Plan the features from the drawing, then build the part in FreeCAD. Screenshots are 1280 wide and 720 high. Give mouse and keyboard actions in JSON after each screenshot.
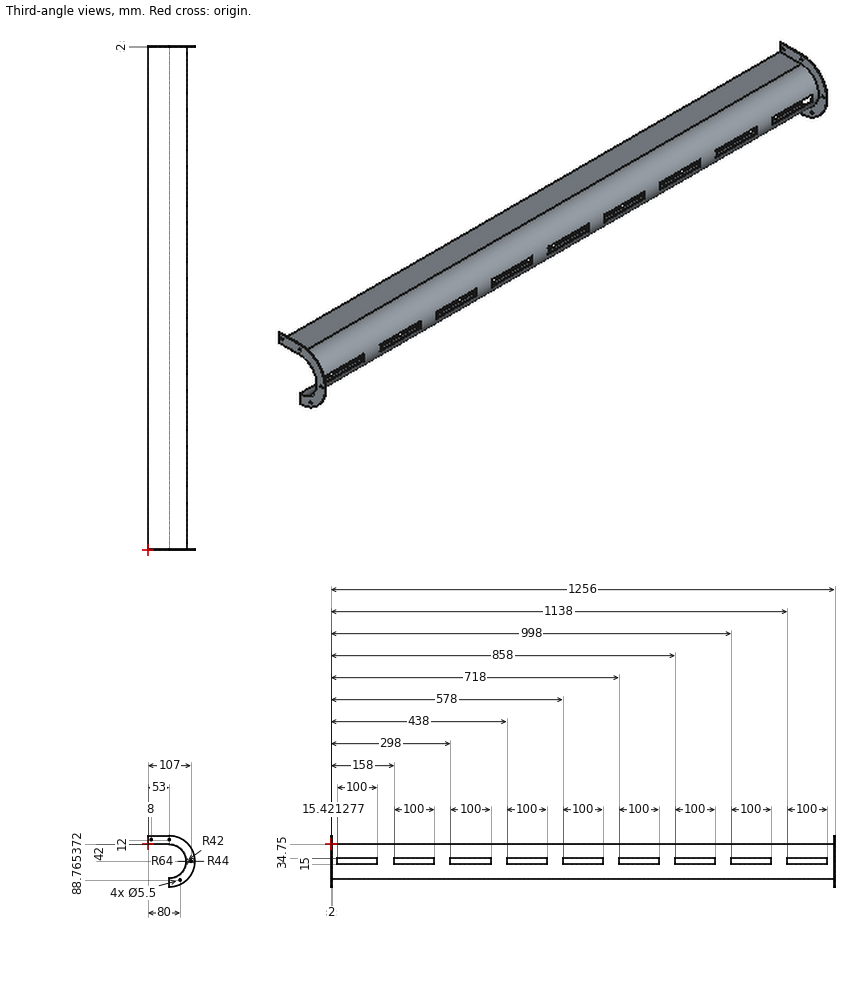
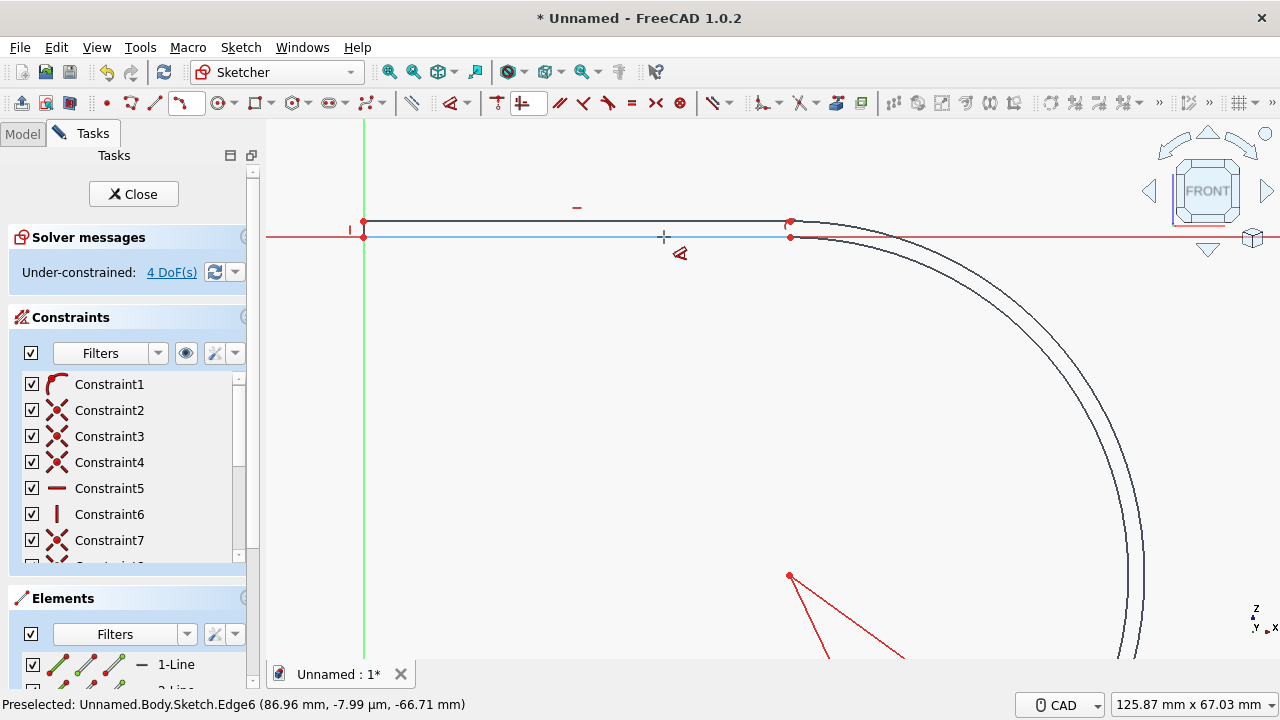
{"action": "left_click", "coordinate": [663, 237]}
{"action": "left_click", "coordinate": [577, 203]}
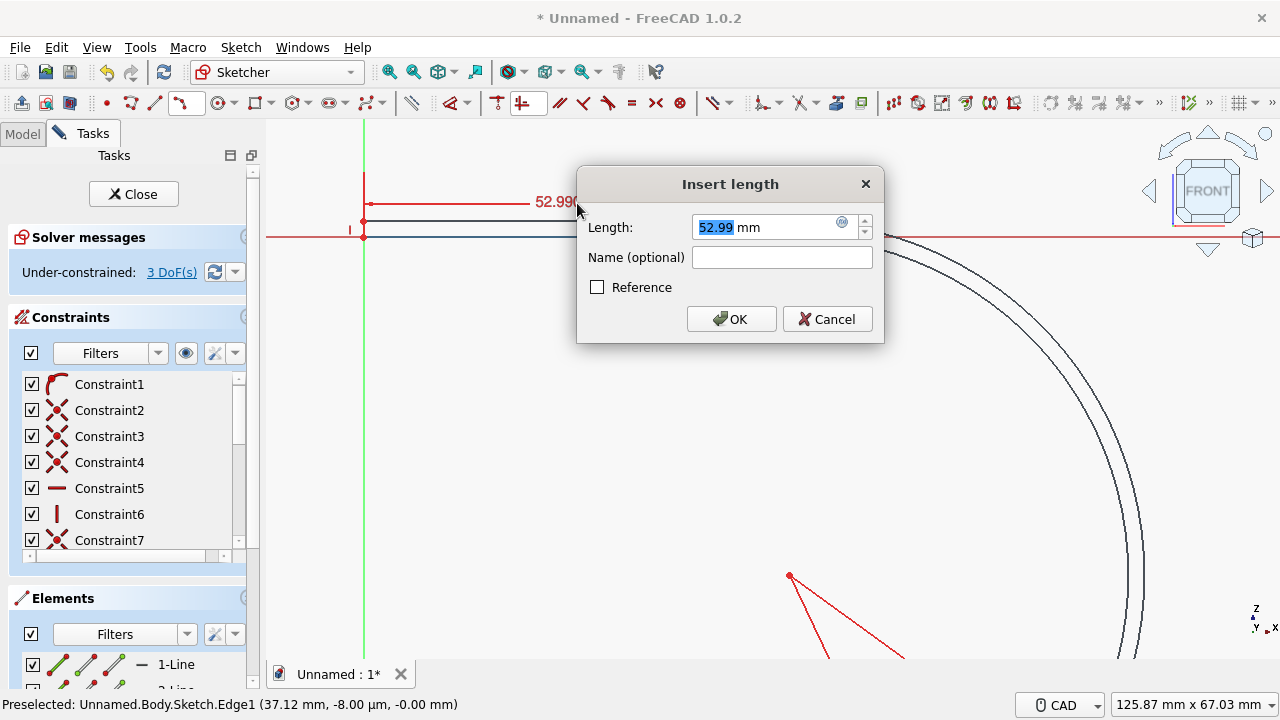
{"action": "type", "text": "53"}
{"action": "key", "text": "Return"}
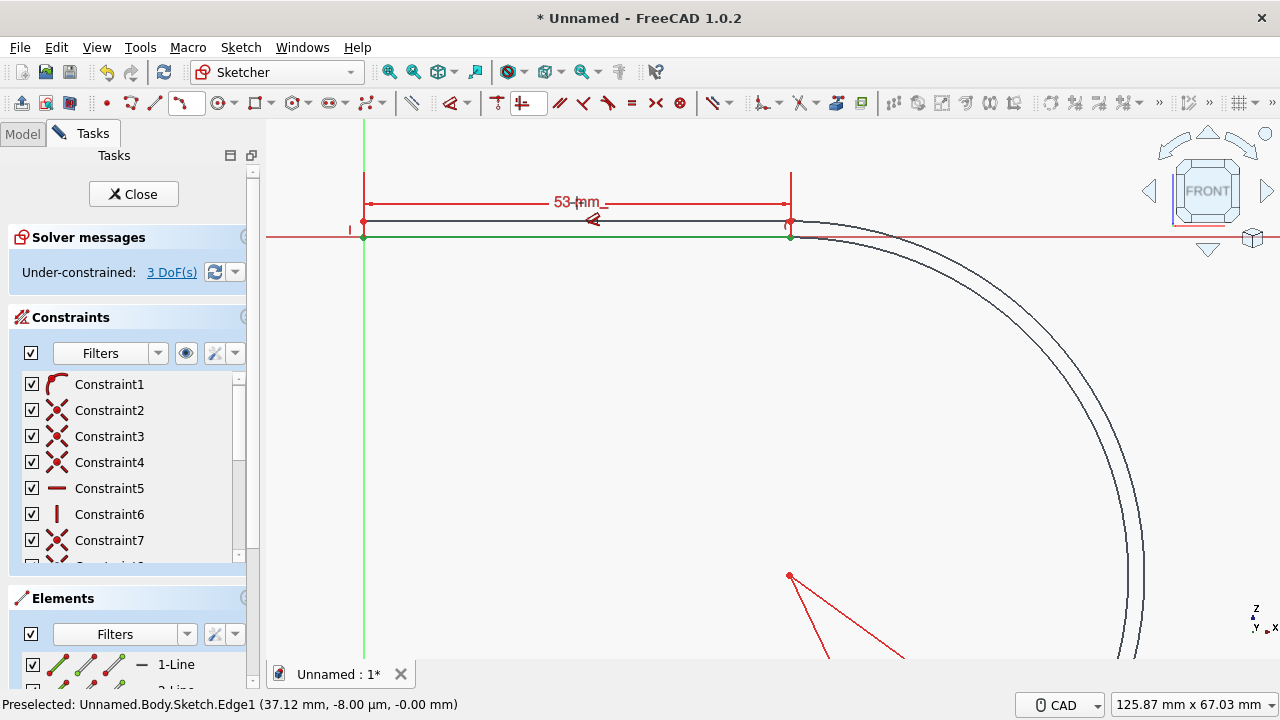
{"action": "left_click", "coordinate": [492, 221]}
{"action": "left_click", "coordinate": [479, 187]}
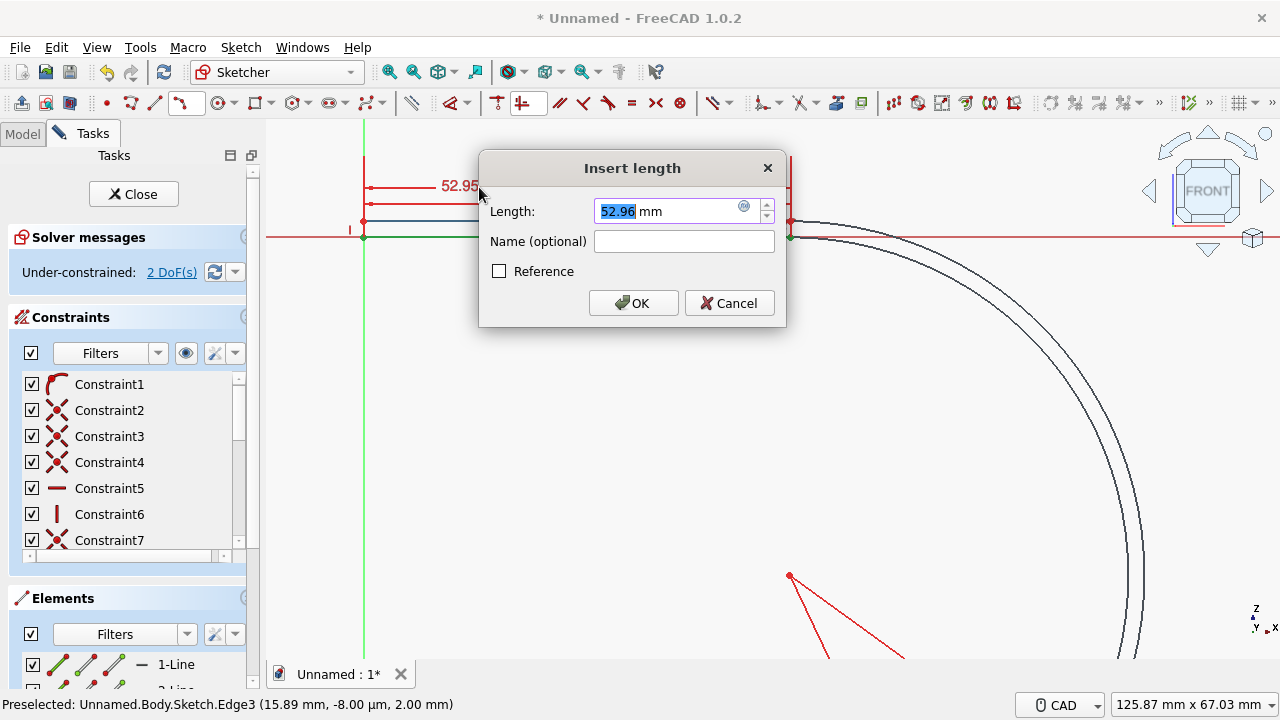
{"action": "type", "text": "53"}
{"action": "key", "text": "Return"}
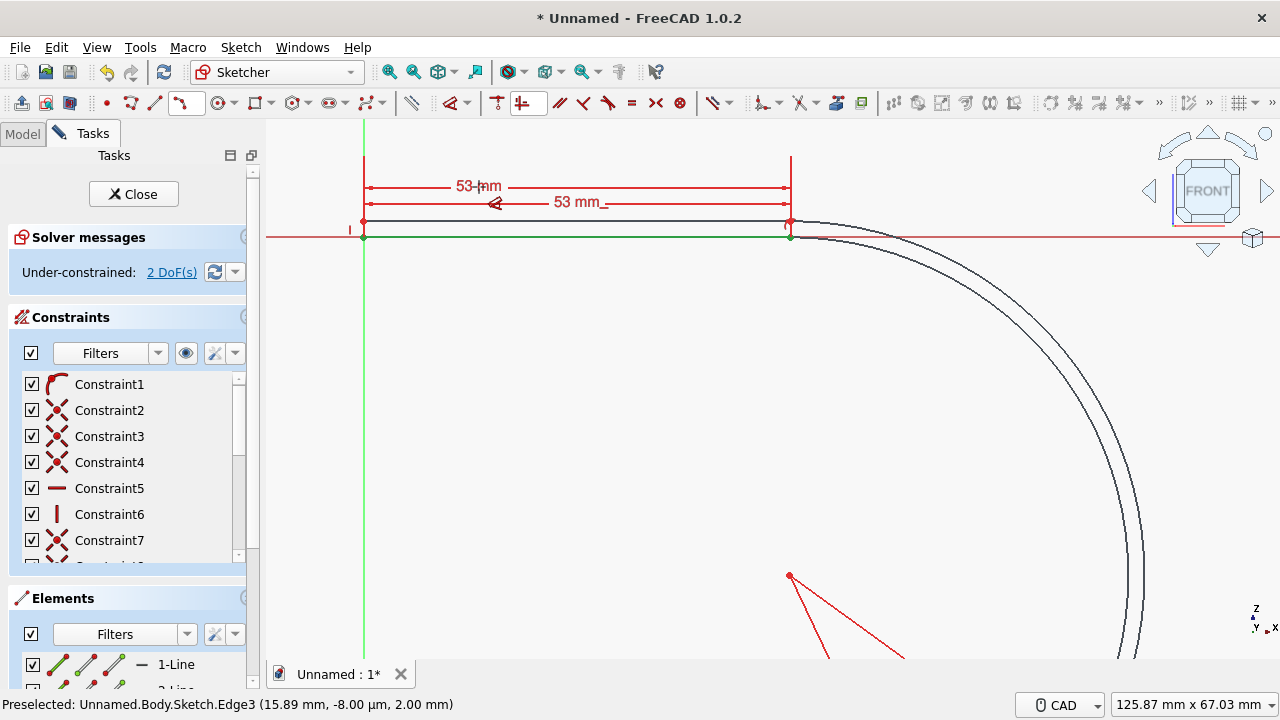
{"action": "scroll", "coordinate": [664, 237], "scroll_direction": "down", "scroll_amount": 4}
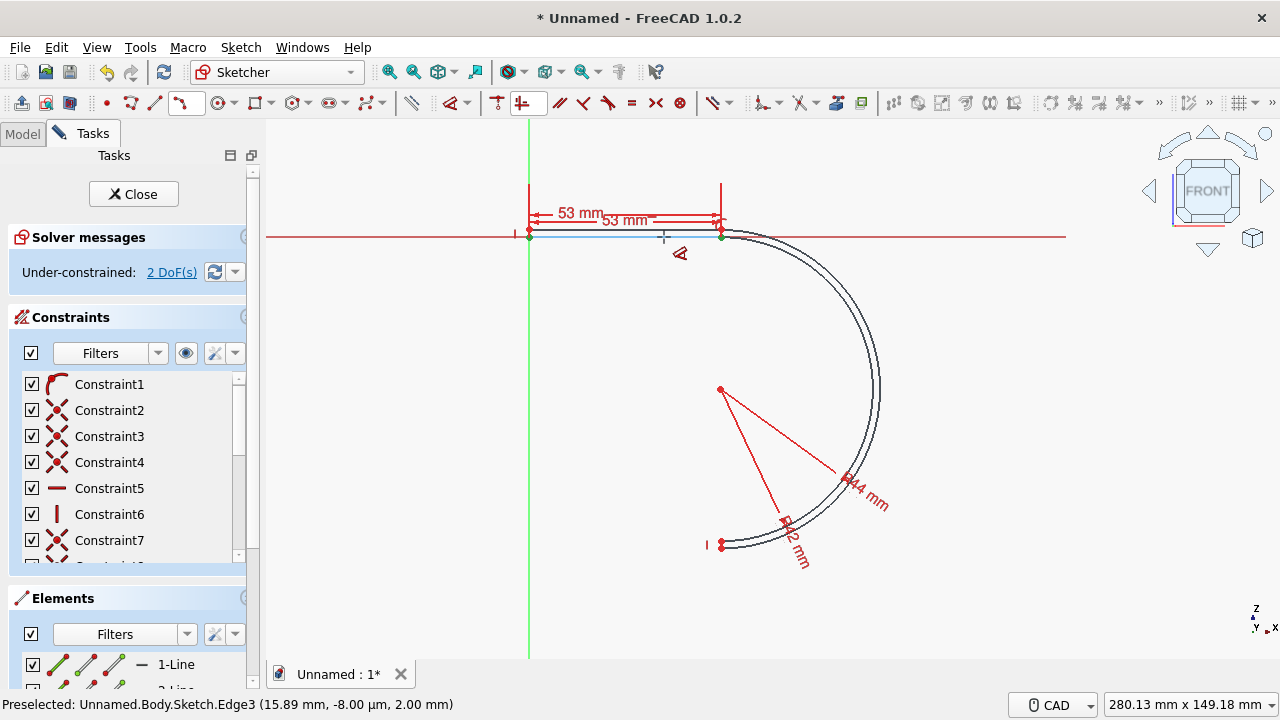
{"action": "scroll", "coordinate": [721, 549], "scroll_direction": "up", "scroll_amount": 3}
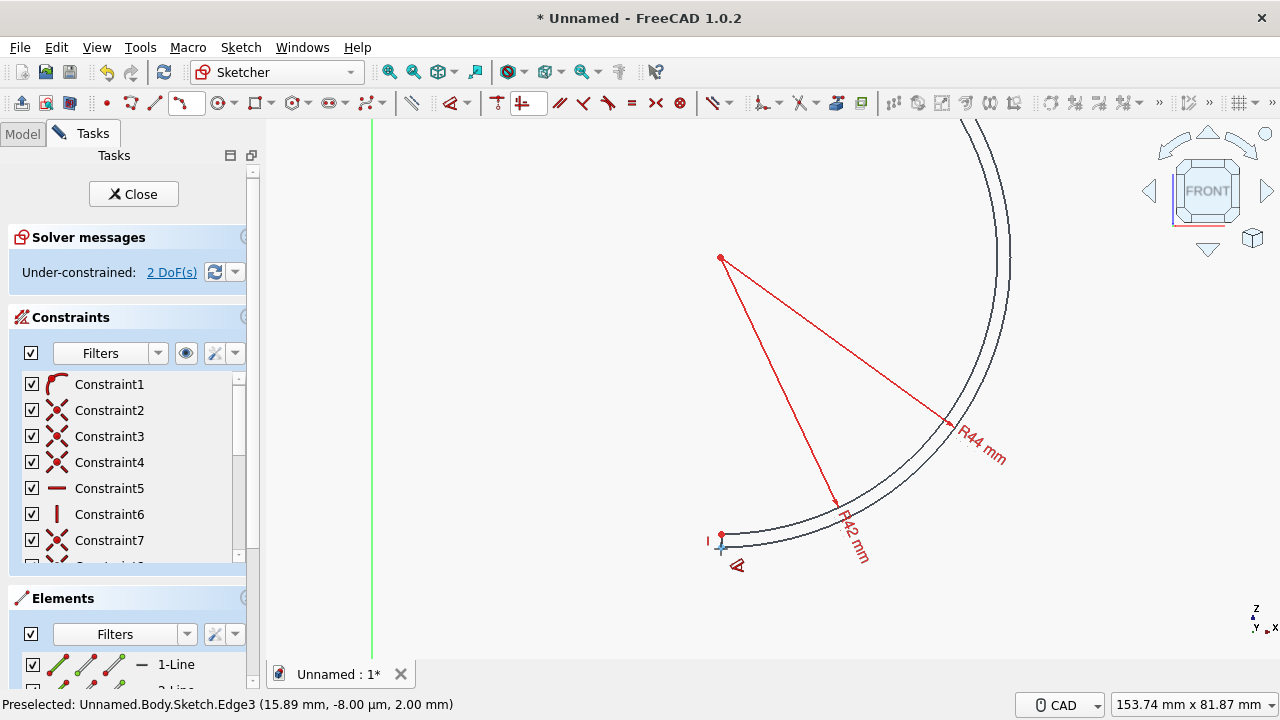
{"action": "left_click", "coordinate": [722, 547]}
{"action": "left_click", "coordinate": [547, 581]}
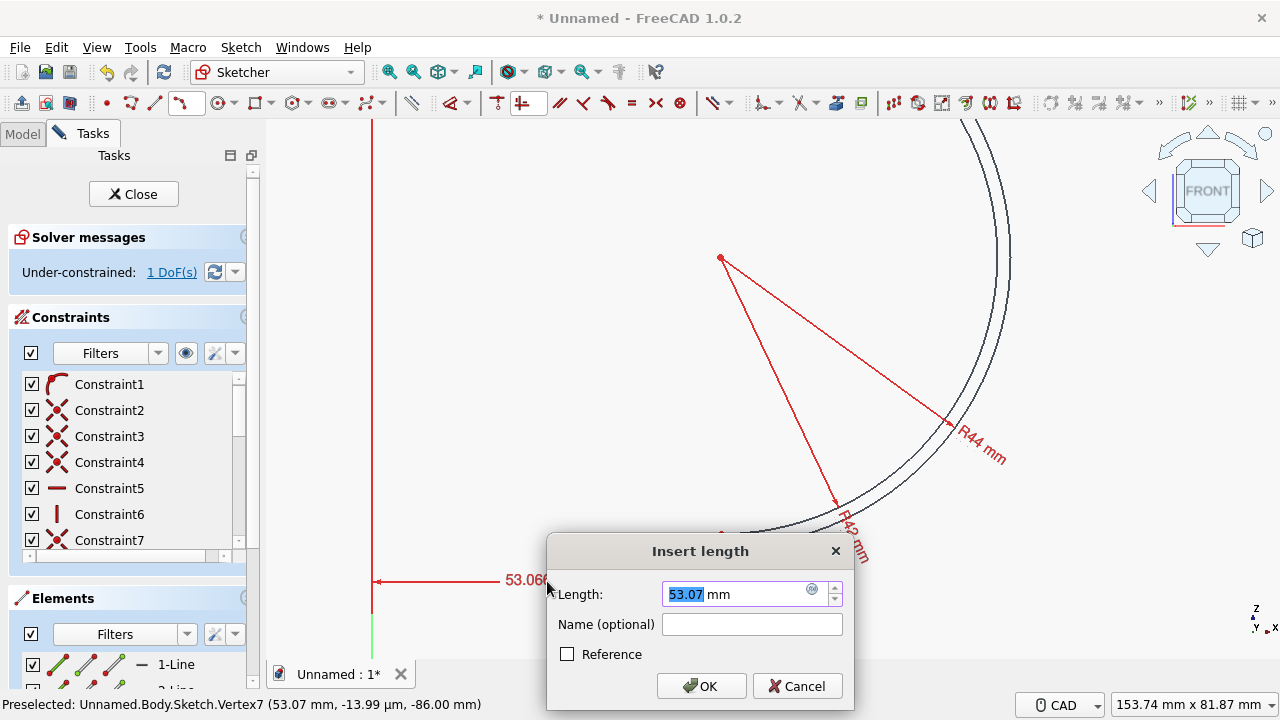
{"action": "type", "text": "53"}
{"action": "key", "text": "Return"}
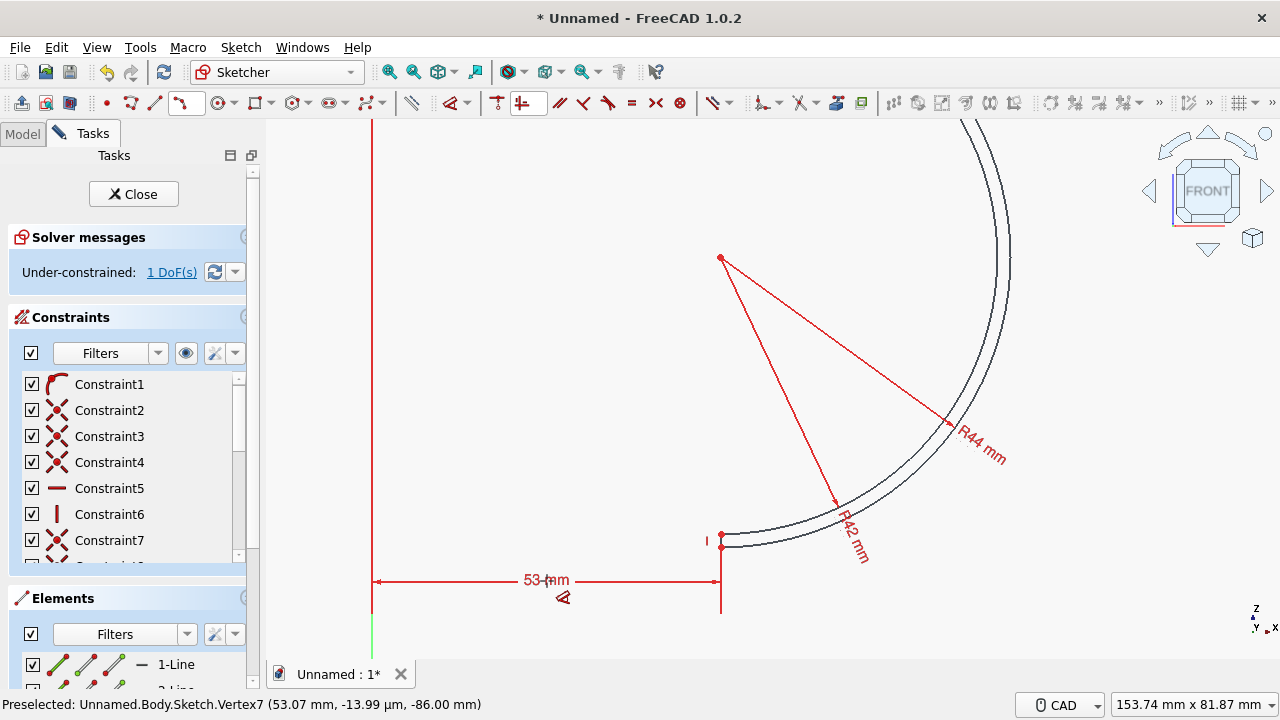
{"action": "left_click", "coordinate": [720, 257]}
{"action": "left_click", "coordinate": [546, 291]}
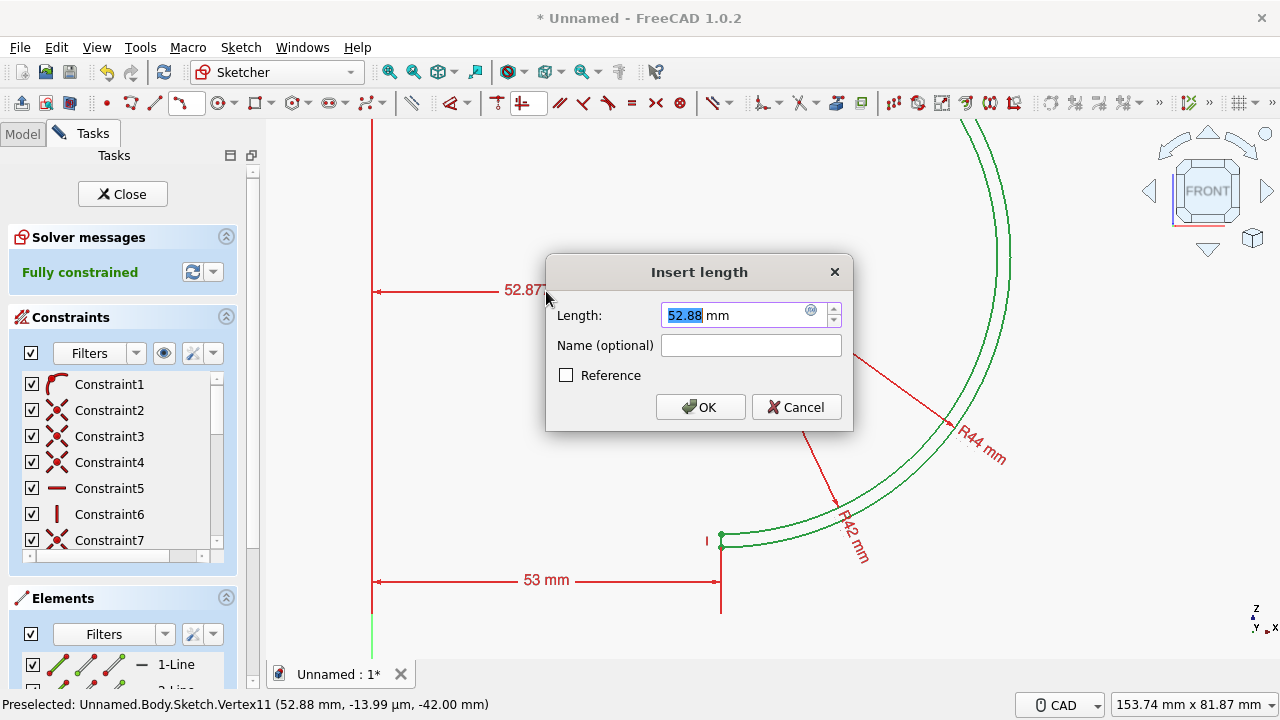
{"action": "type", "text": "53"}
{"action": "key", "text": "Return"}
{"action": "key", "text": "Escape"}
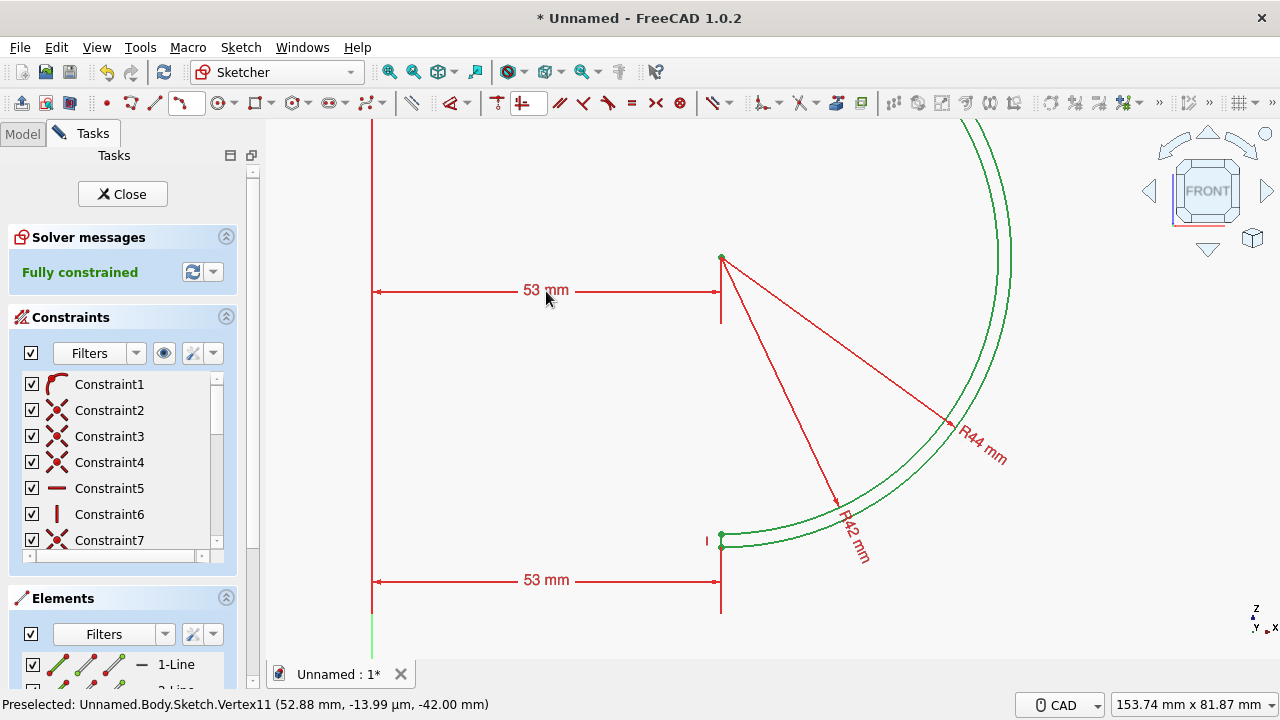
{"action": "left_click", "coordinate": [123, 194]}